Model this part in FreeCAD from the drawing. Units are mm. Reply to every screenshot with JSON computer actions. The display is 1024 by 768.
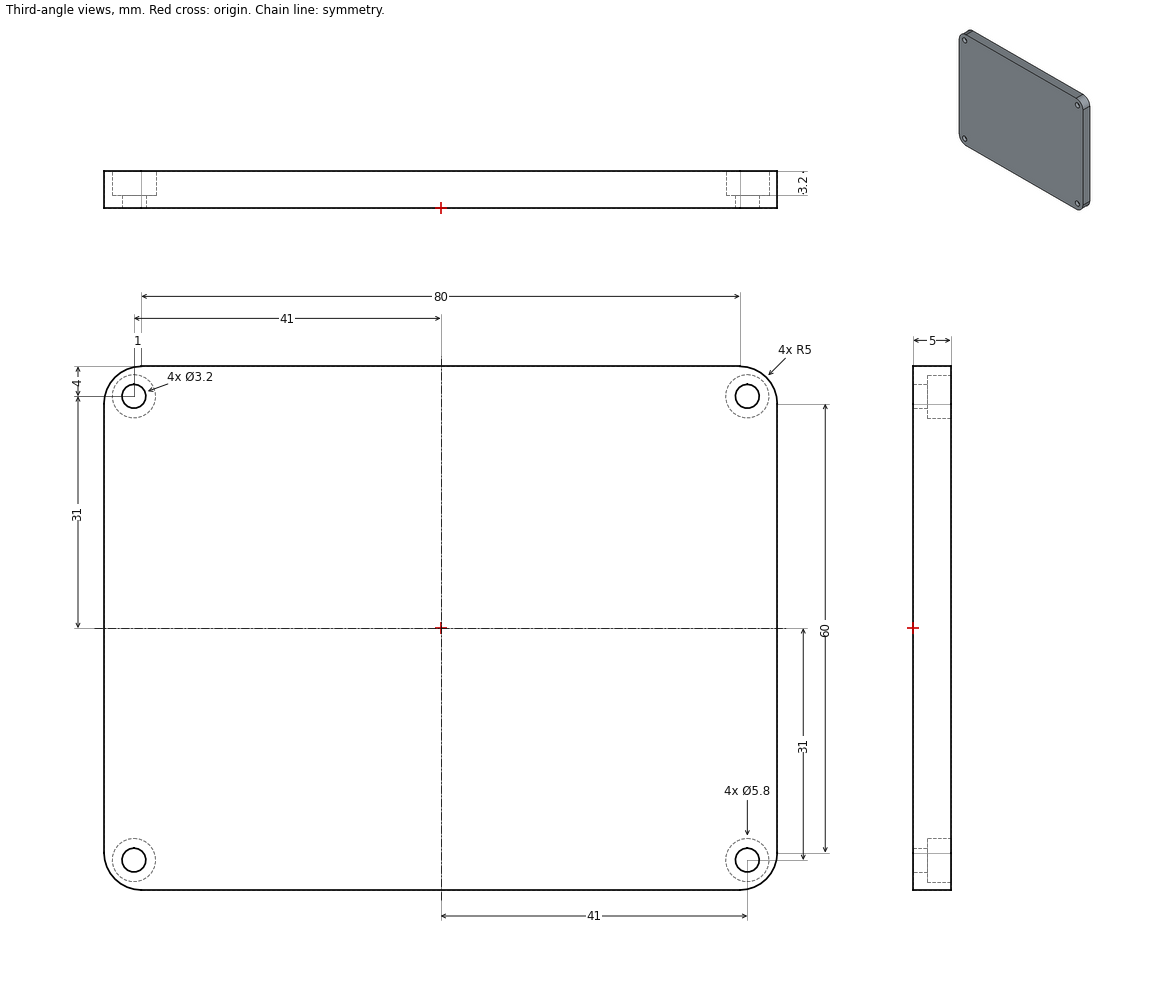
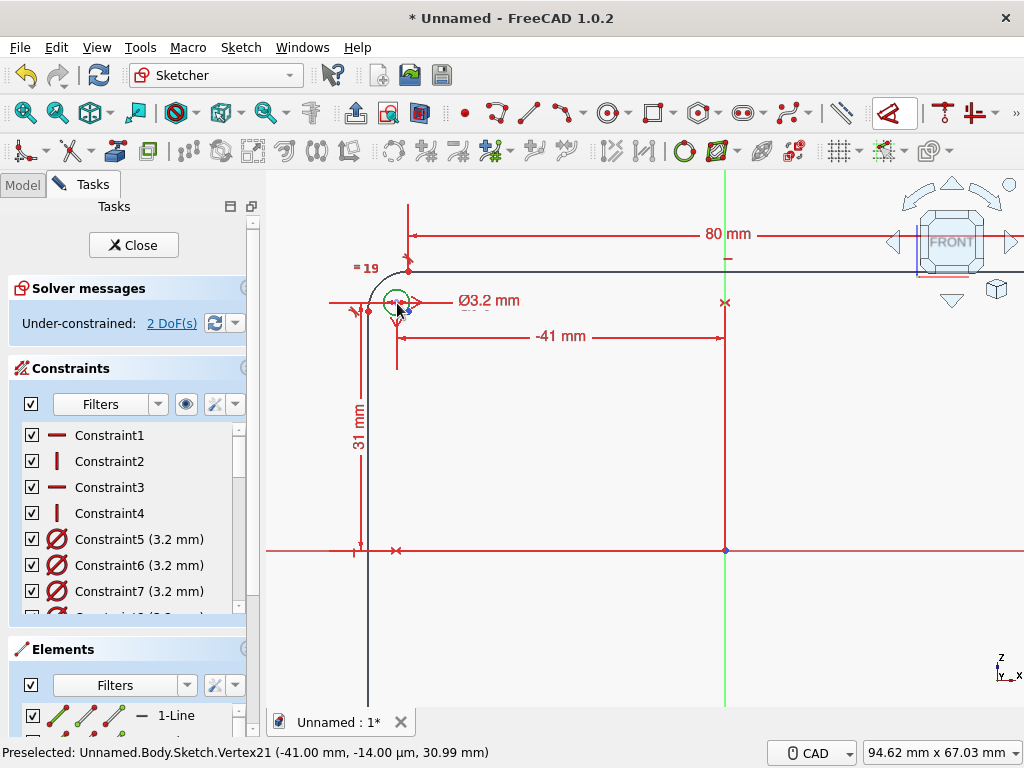
{"action": "scroll", "coordinate": [408, 272], "scroll_direction": "up", "scroll_amount": 9}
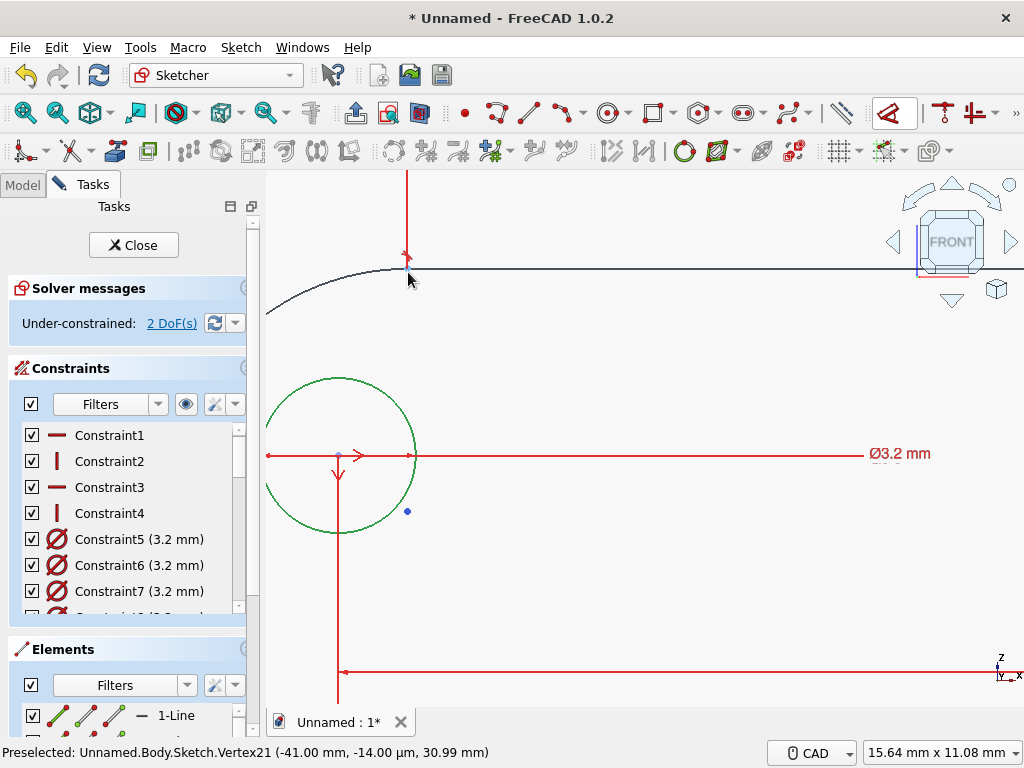
{"action": "left_click", "coordinate": [407, 269]}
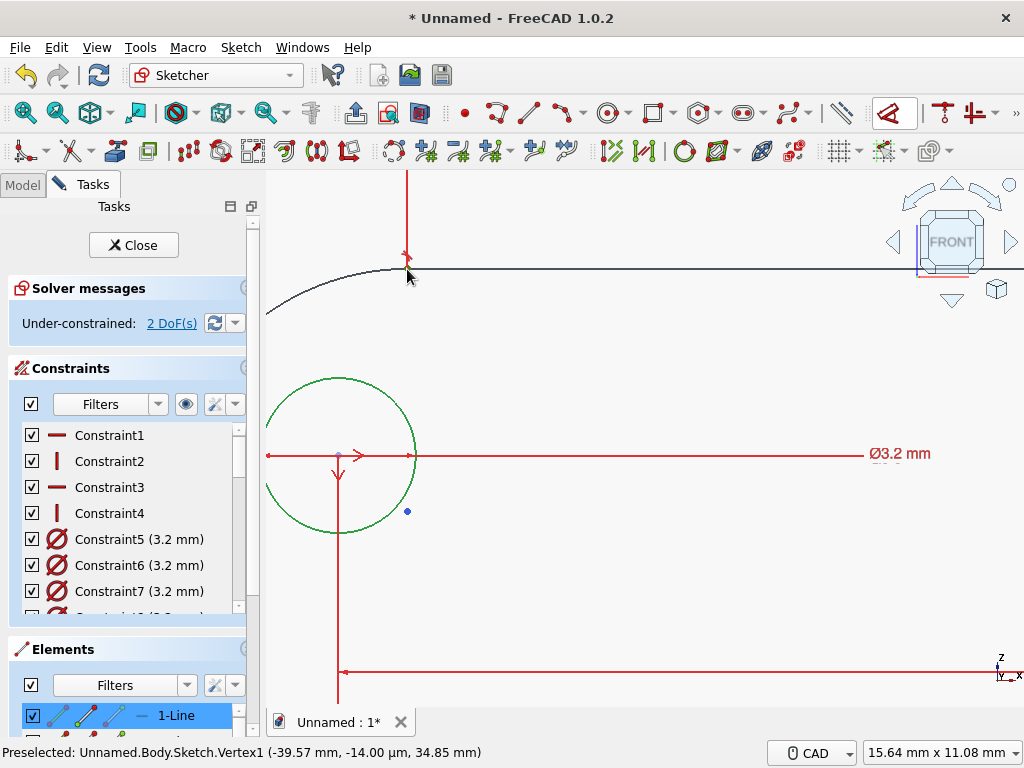
{"action": "left_click", "coordinate": [338, 456]}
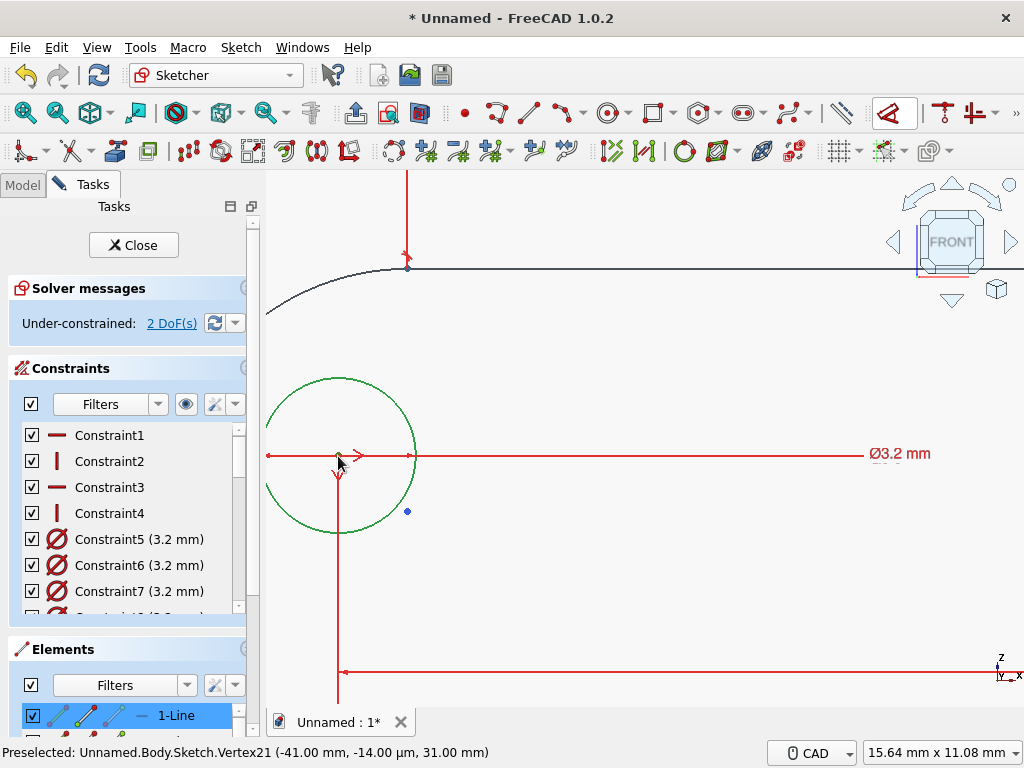
{"action": "left_click", "coordinate": [912, 114]}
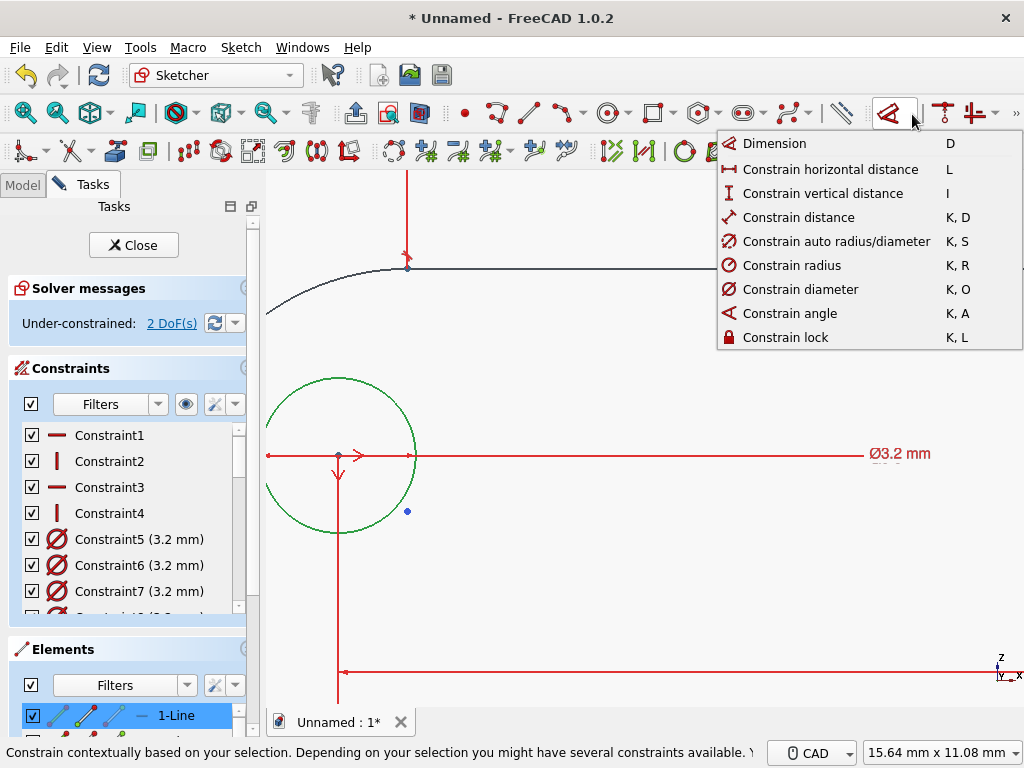
{"action": "left_click", "coordinate": [870, 169]}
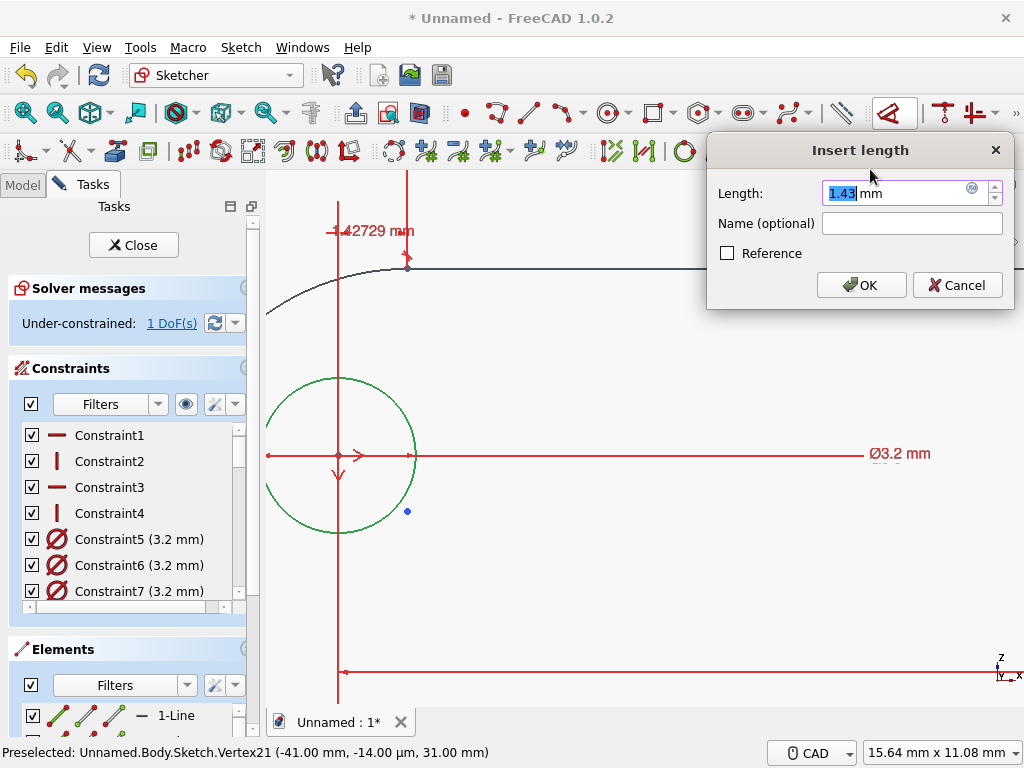
{"action": "type", "text": "1"}
{"action": "key", "text": "Return"}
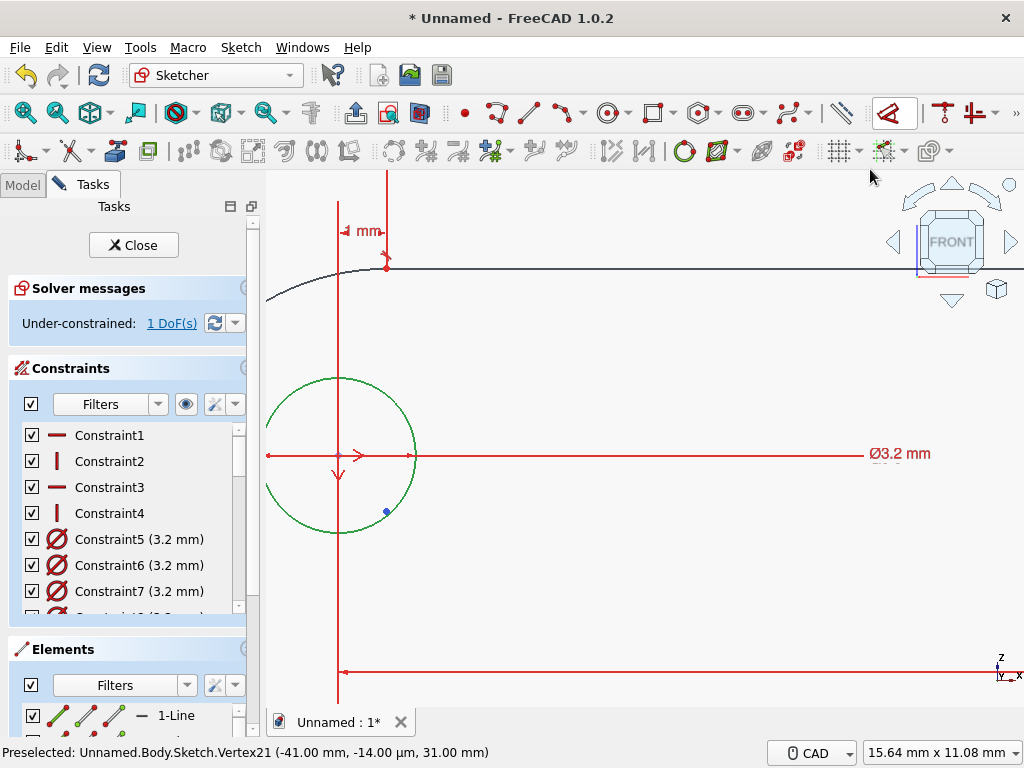
{"action": "scroll", "coordinate": [402, 287], "scroll_direction": "down", "scroll_amount": 12}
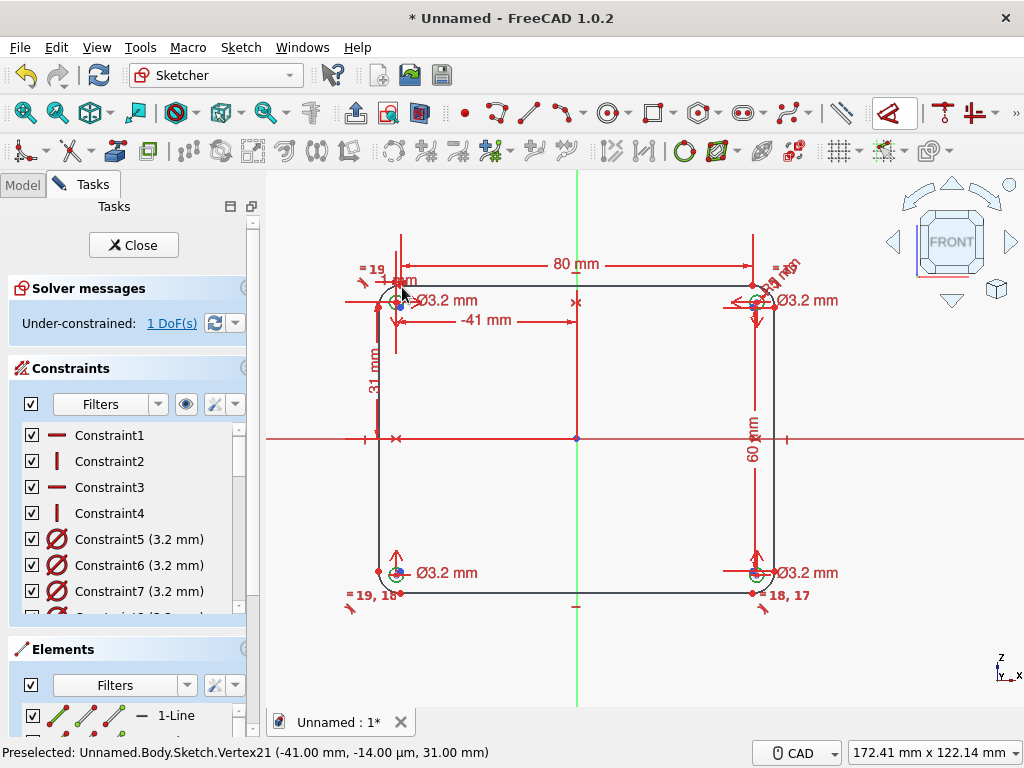
{"action": "scroll", "coordinate": [401, 286], "scroll_direction": "up", "scroll_amount": 5}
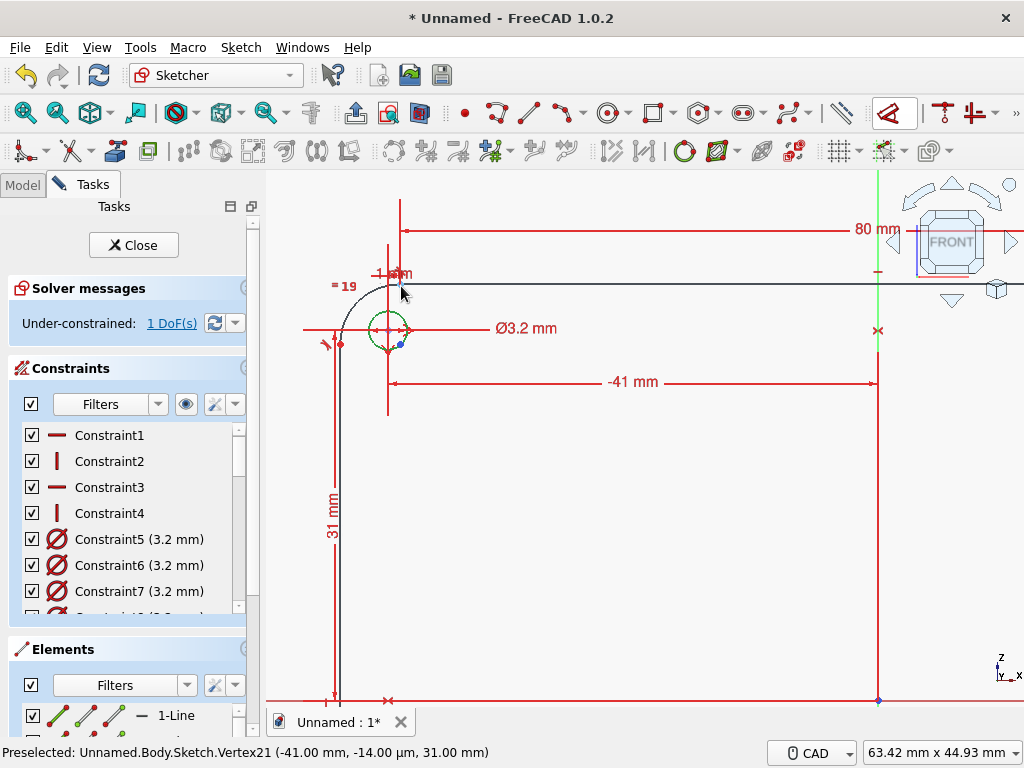
{"action": "left_click", "coordinate": [400, 284]}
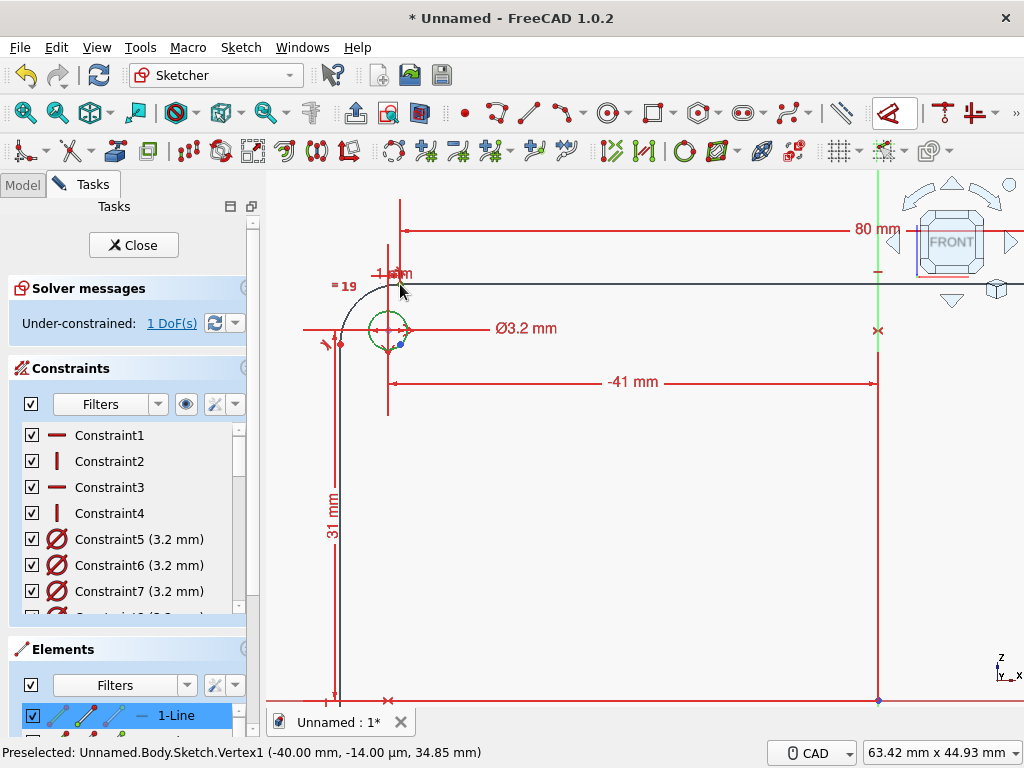
{"action": "left_click", "coordinate": [388, 330]}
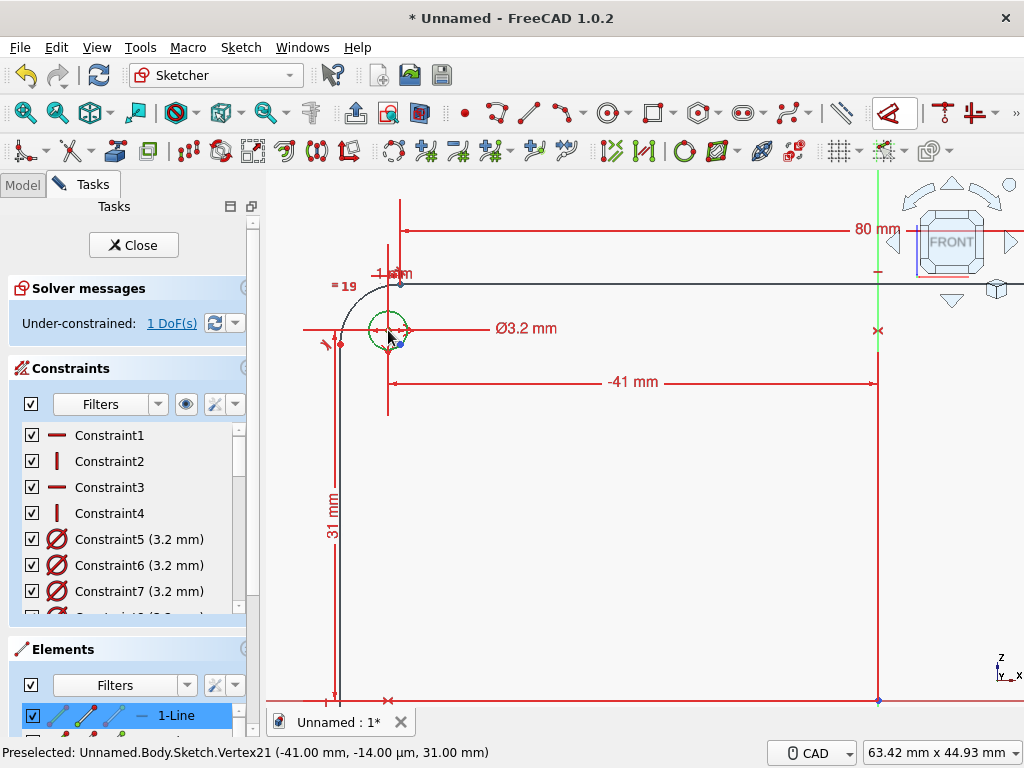
{"action": "key", "text": "i"}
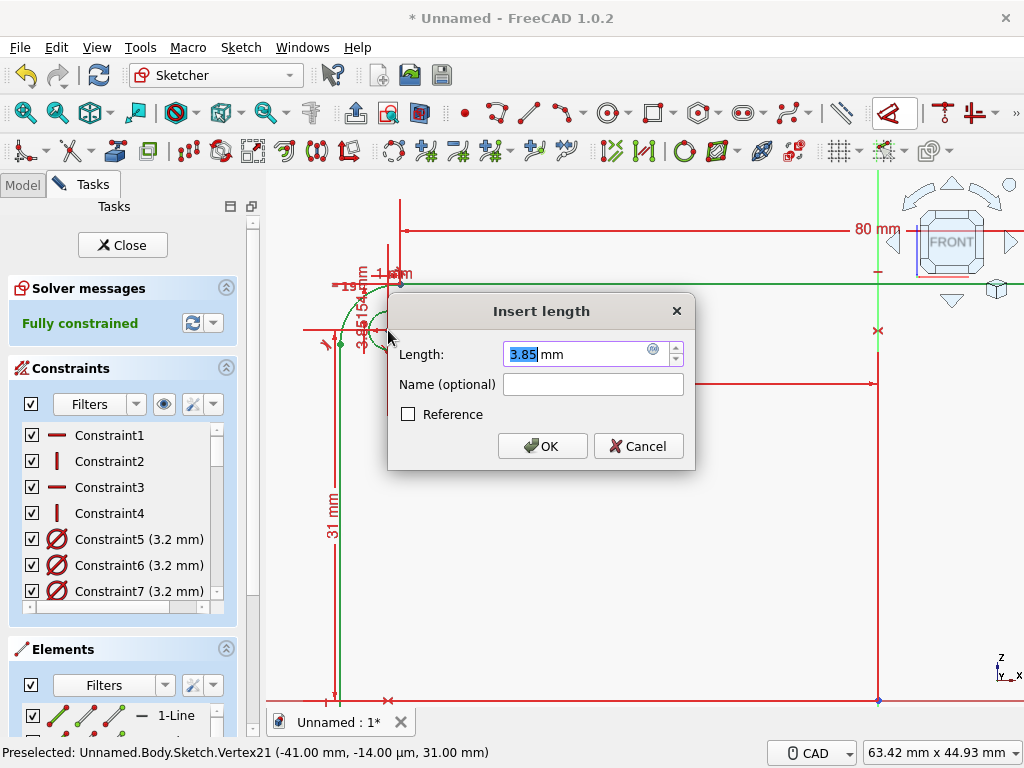
{"action": "type", "text": "4"}
{"action": "key", "text": "Return"}